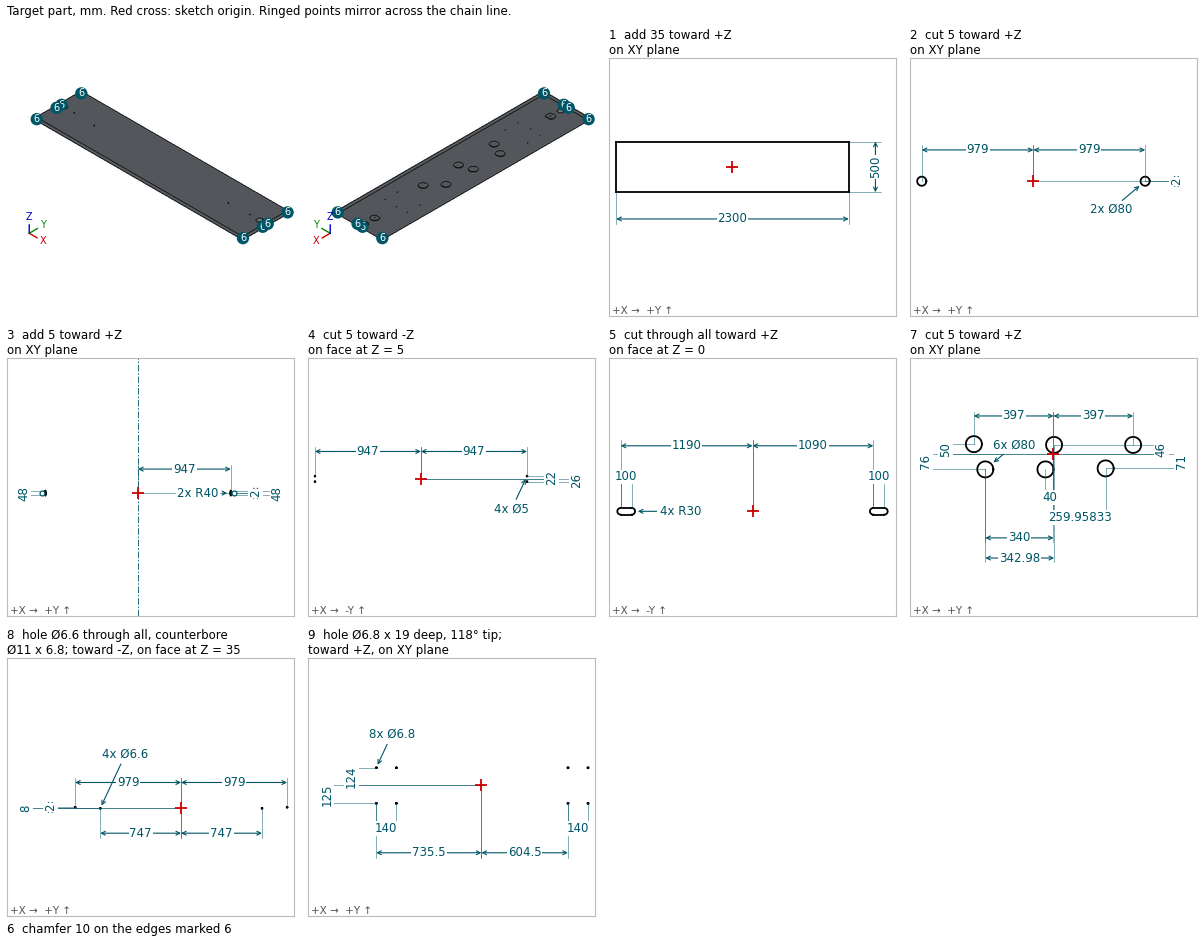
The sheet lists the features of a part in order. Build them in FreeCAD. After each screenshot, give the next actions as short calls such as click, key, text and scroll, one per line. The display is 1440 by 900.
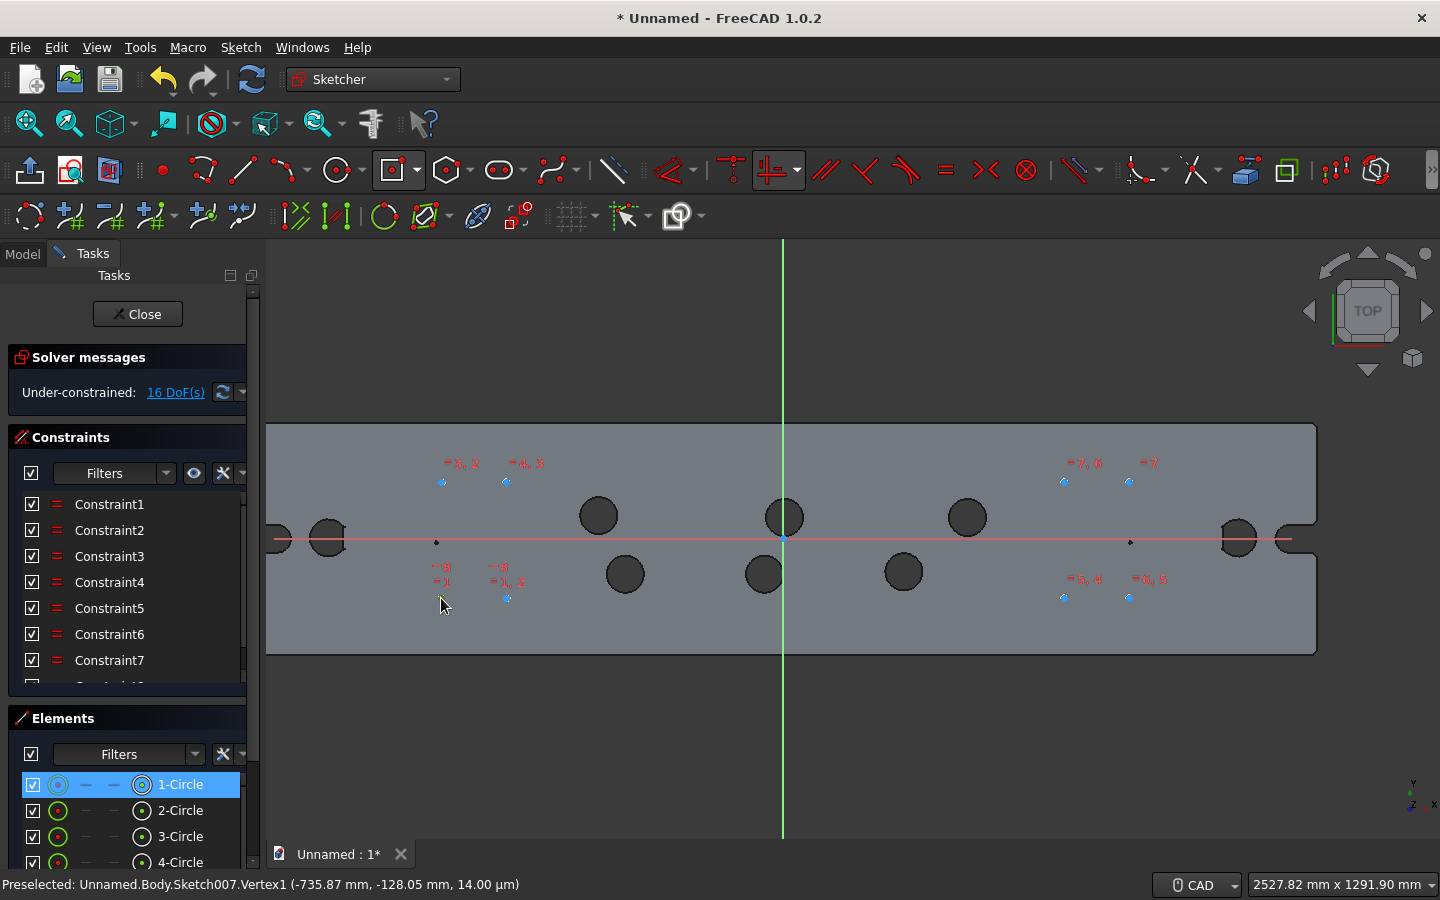
click(442, 483)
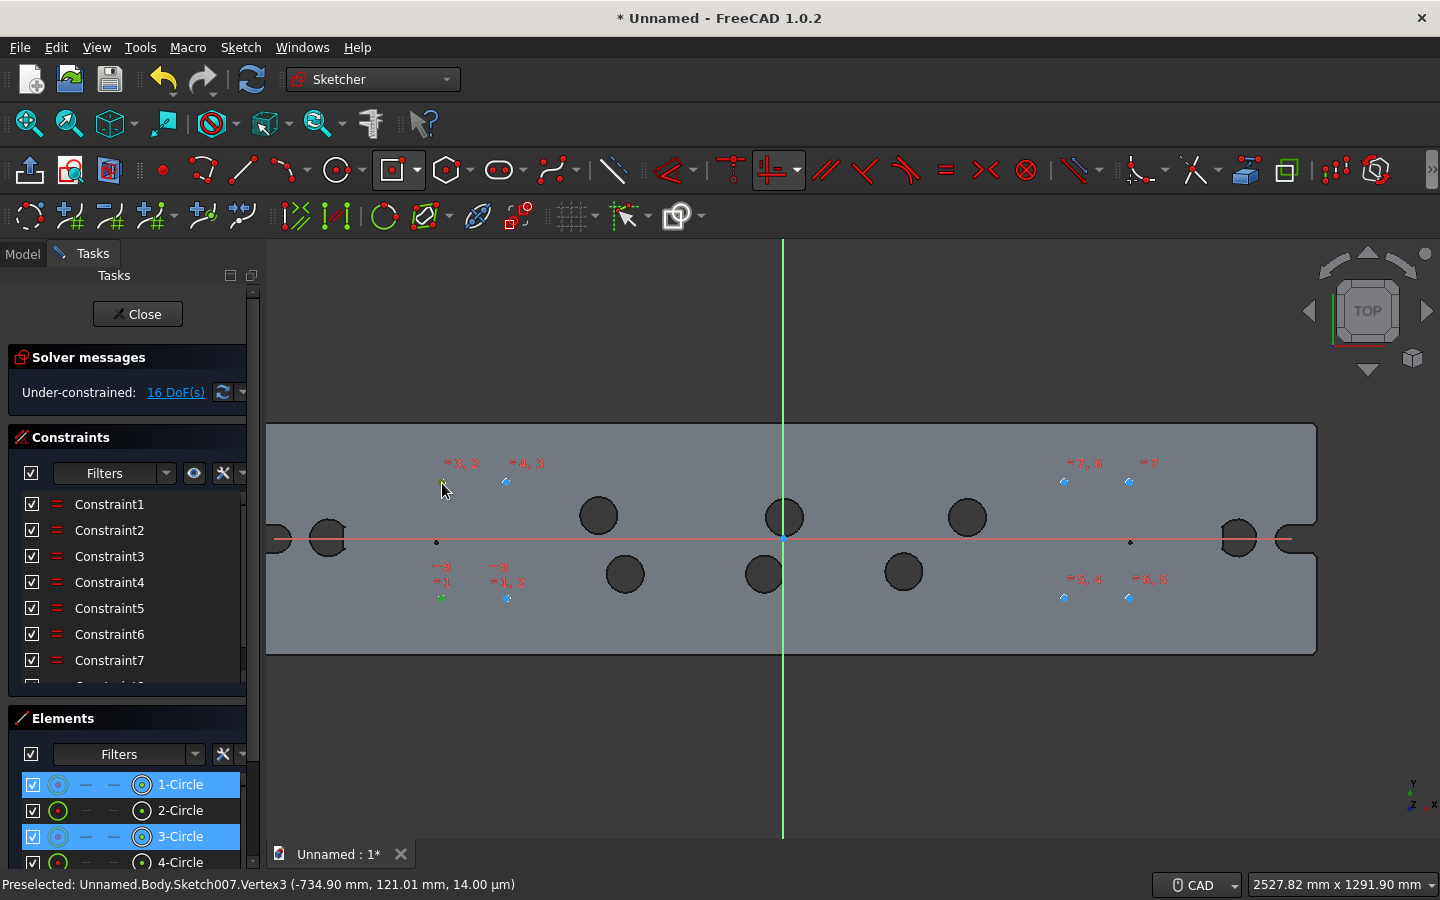
click(800, 170)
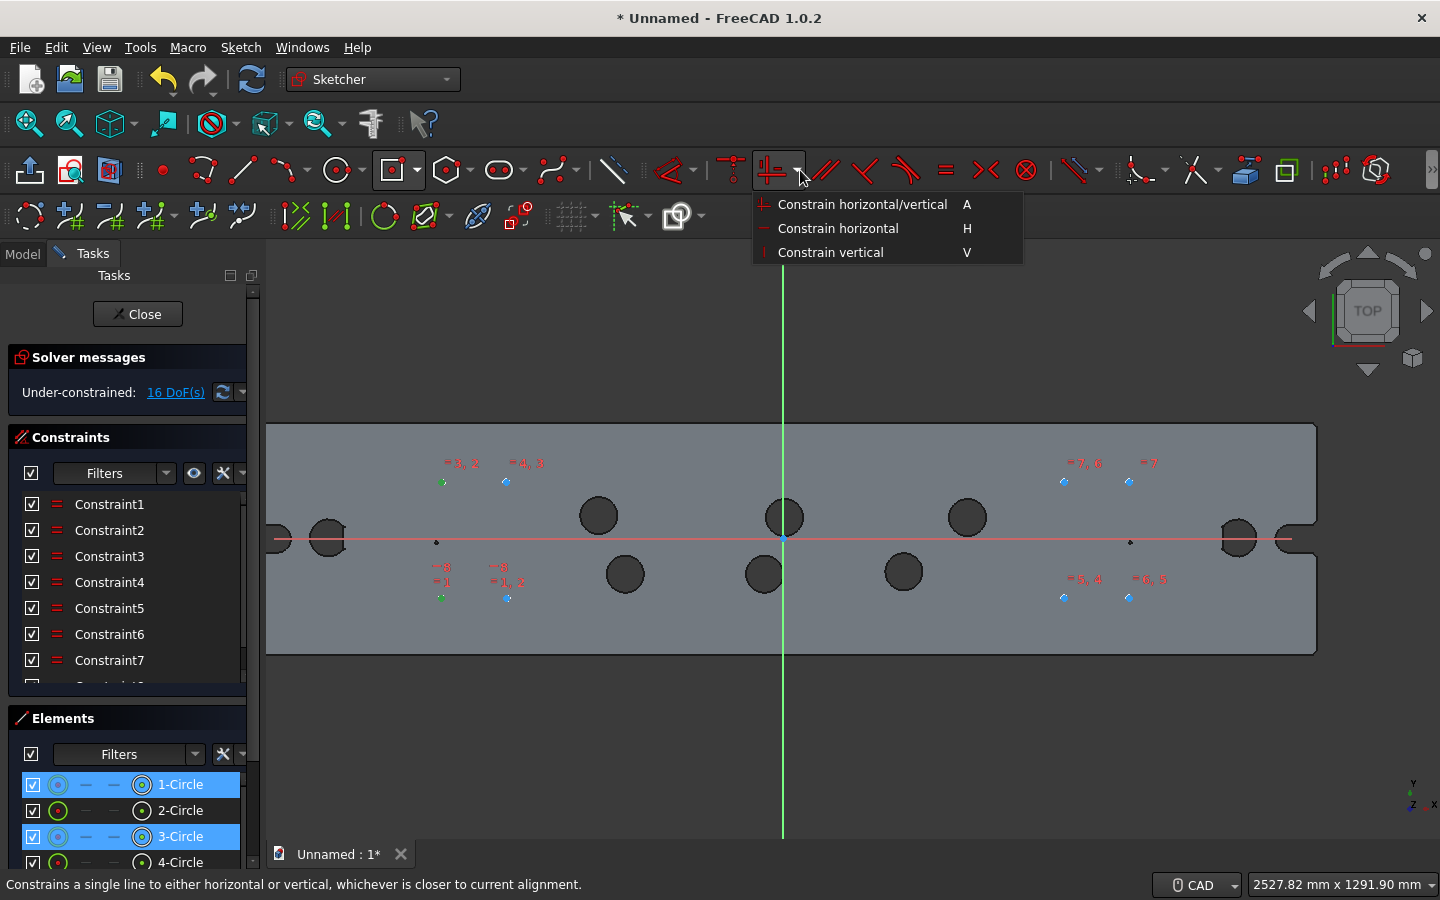
click(888, 252)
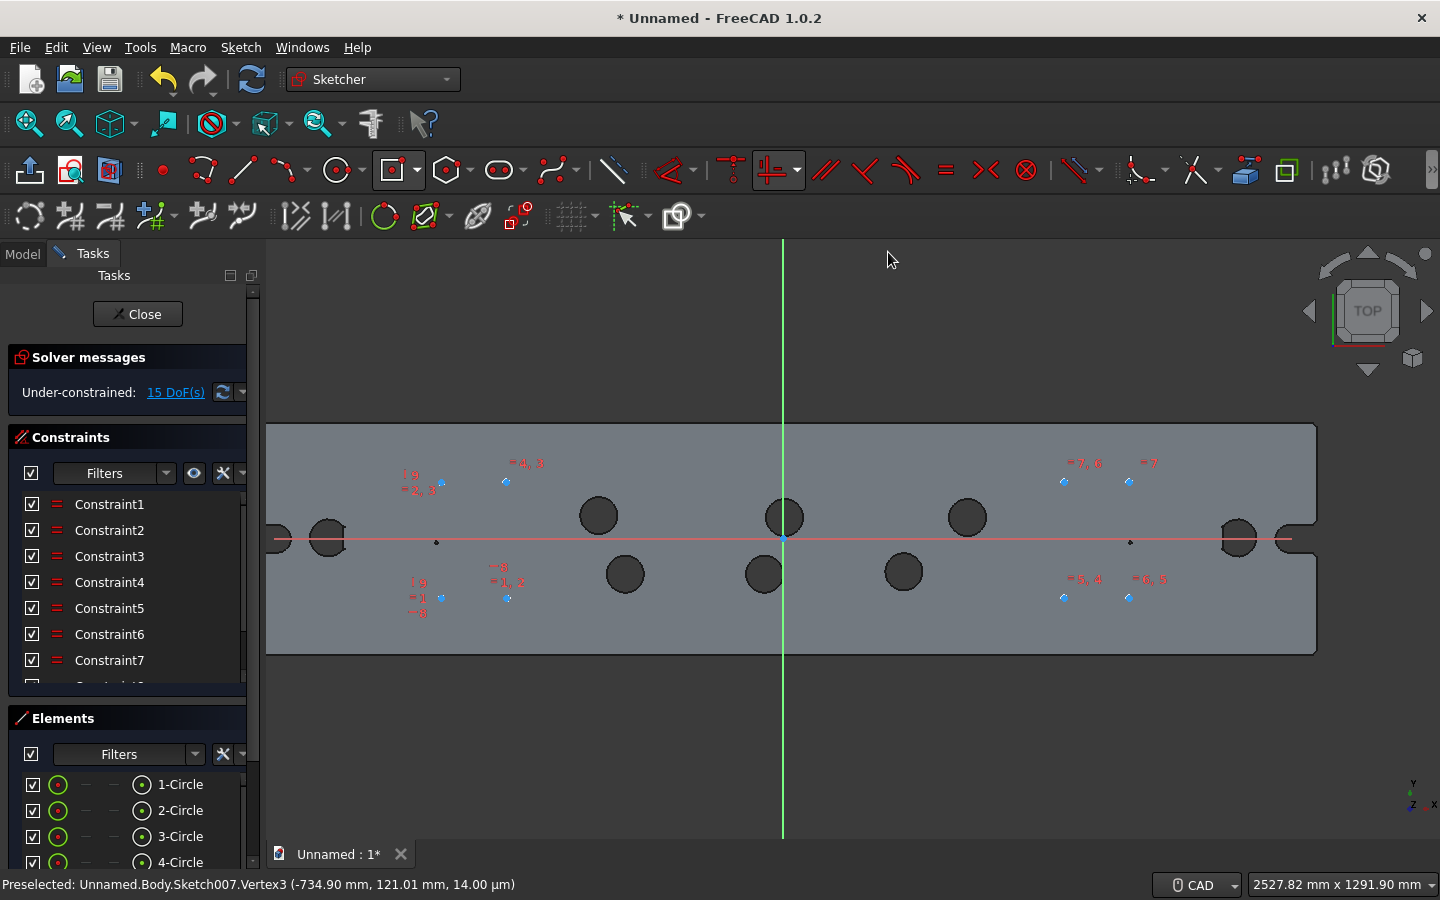
click(507, 598)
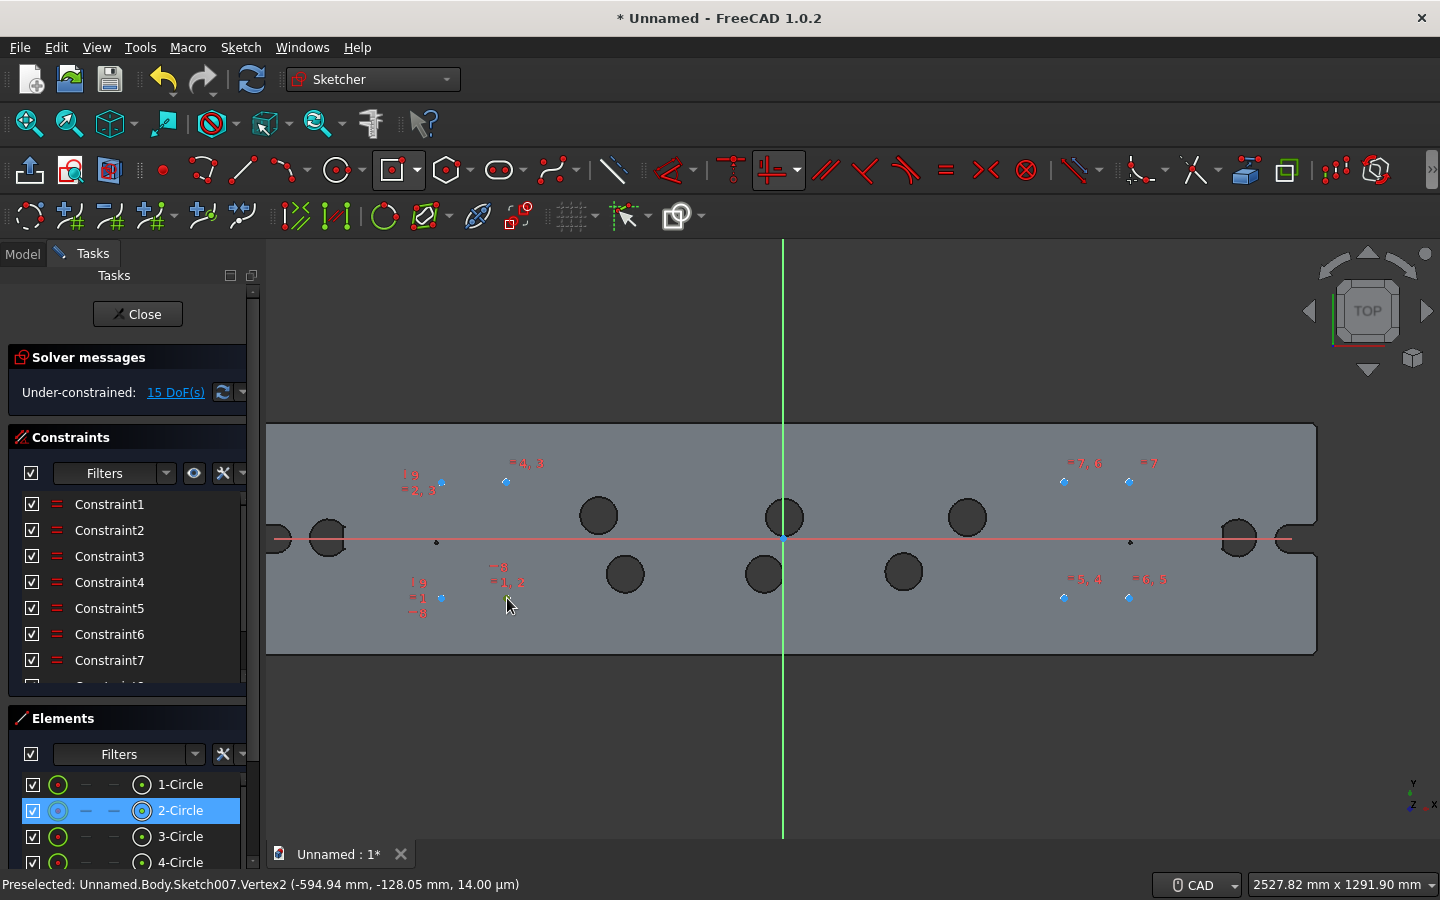
click(506, 482)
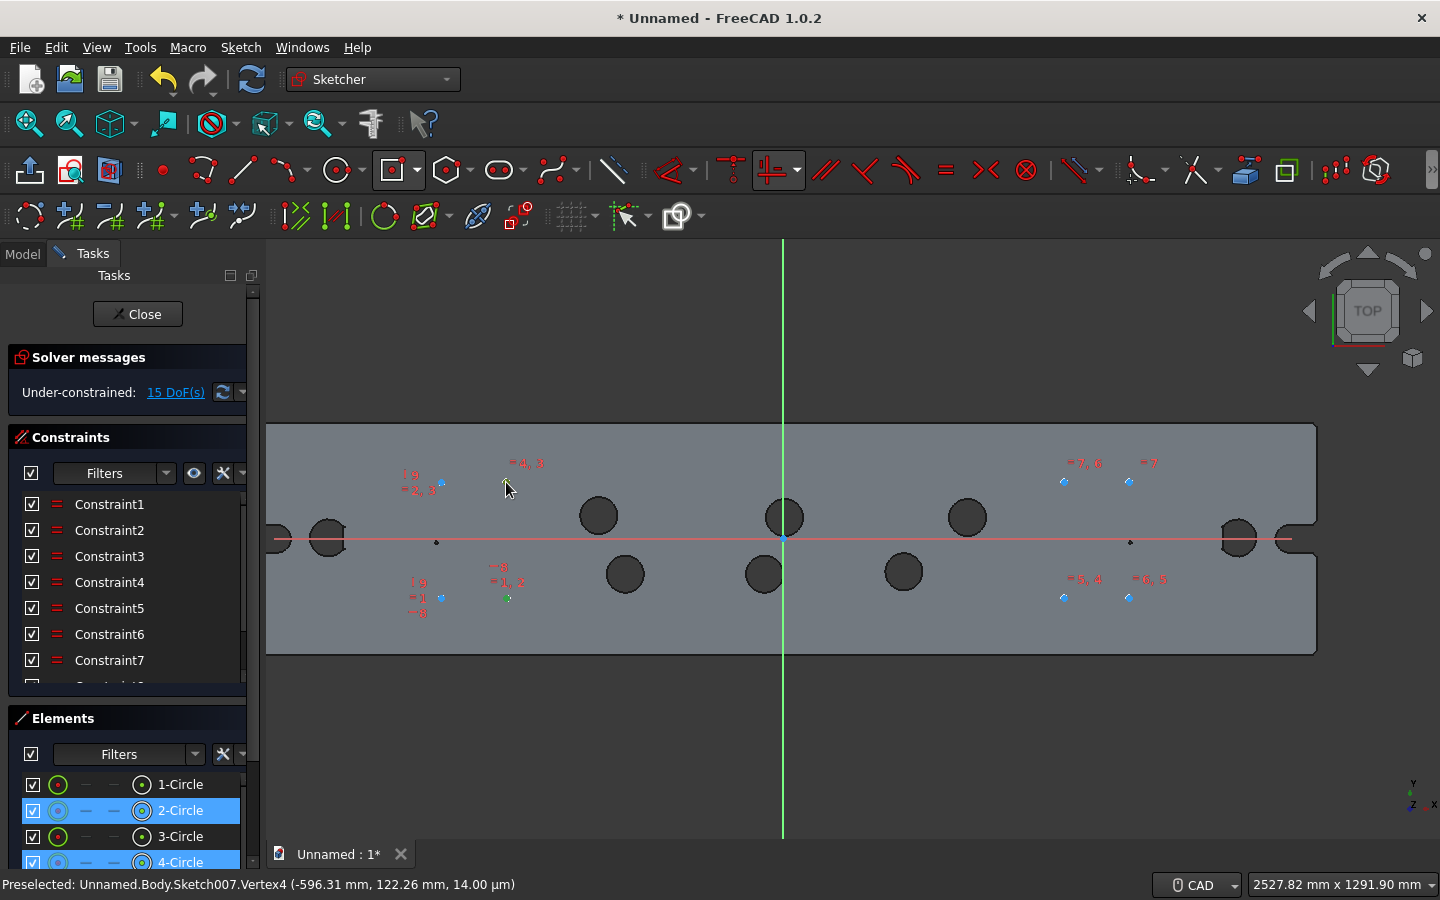
click(800, 170)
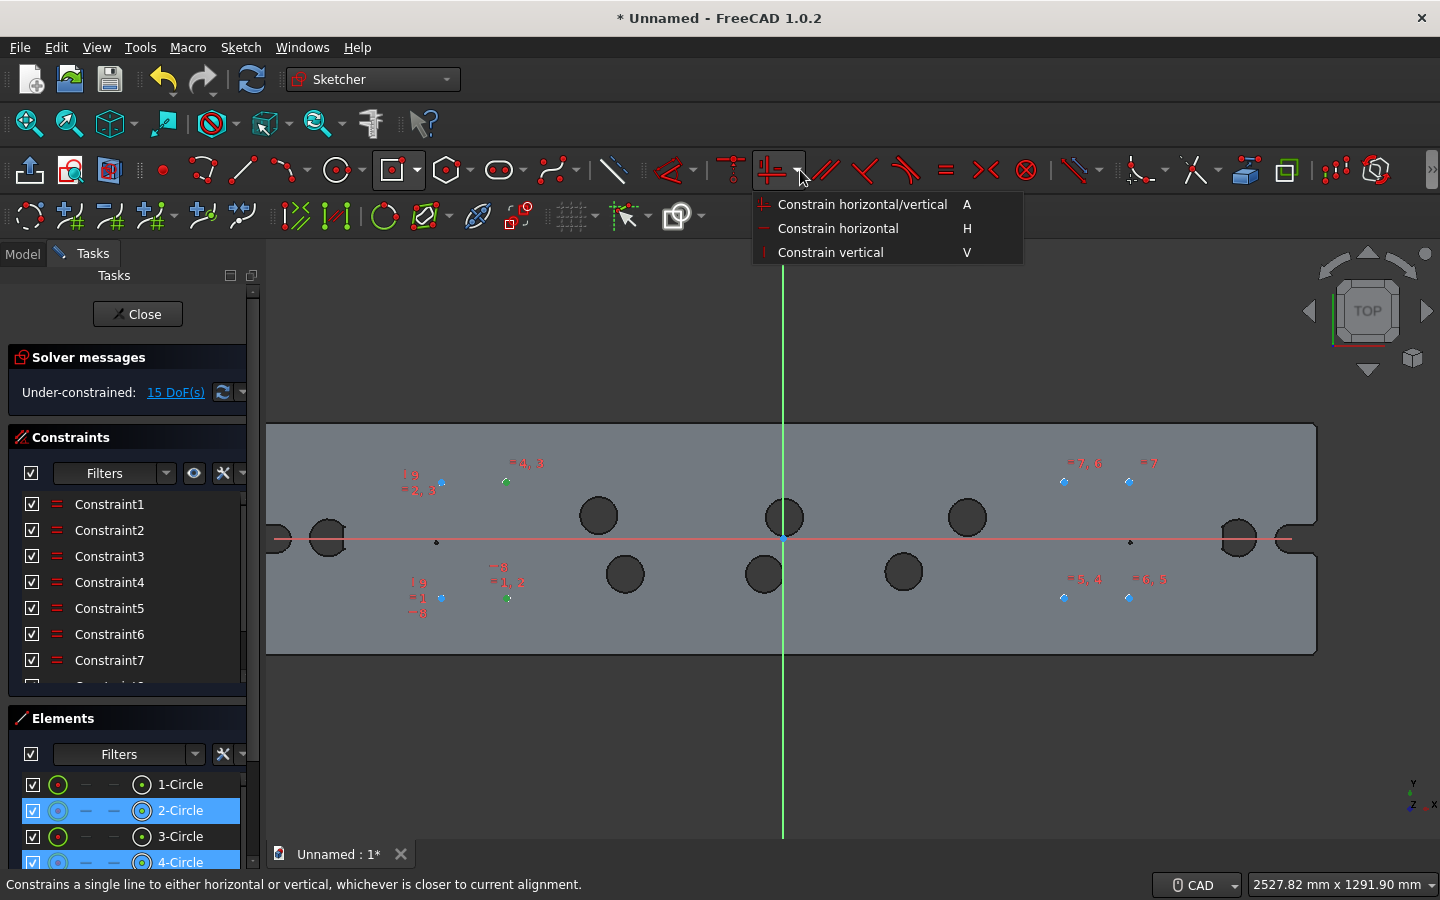
click(888, 252)